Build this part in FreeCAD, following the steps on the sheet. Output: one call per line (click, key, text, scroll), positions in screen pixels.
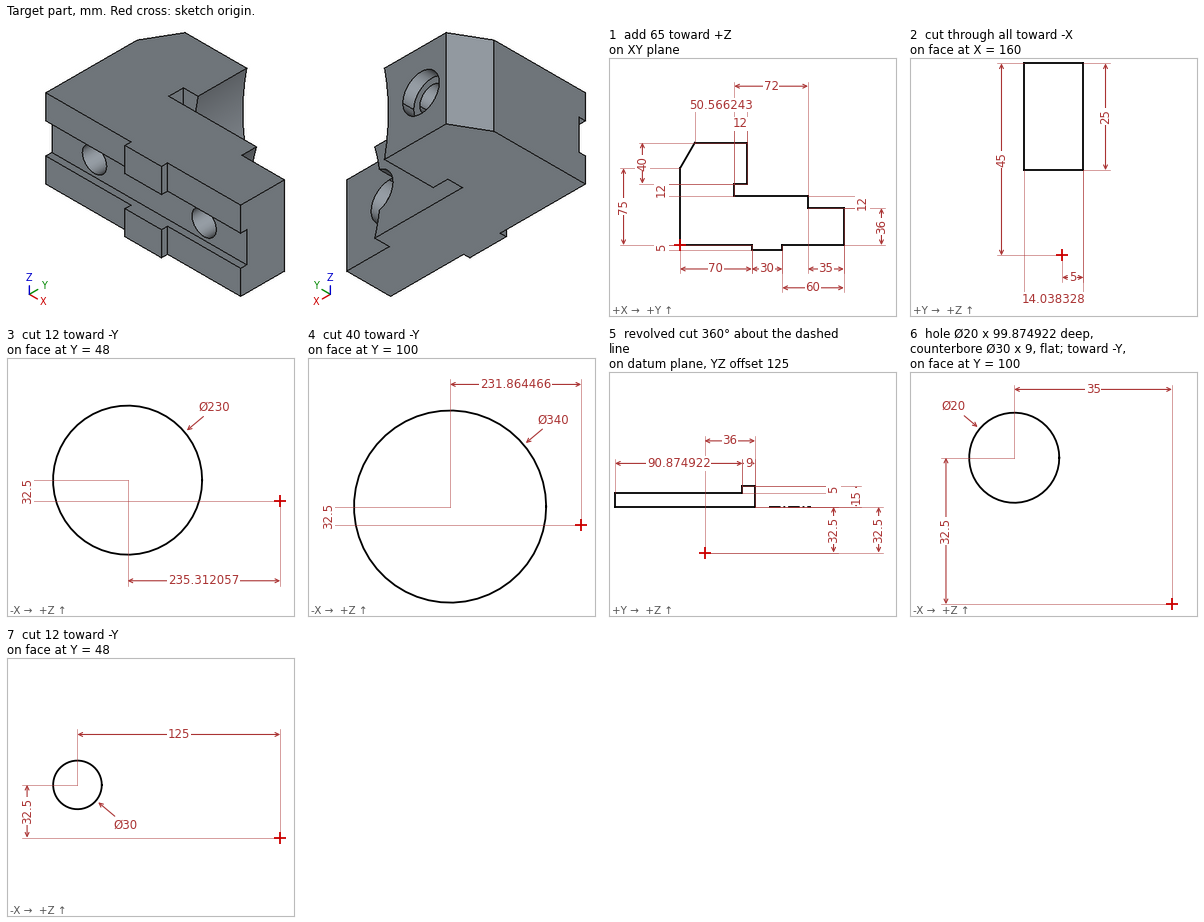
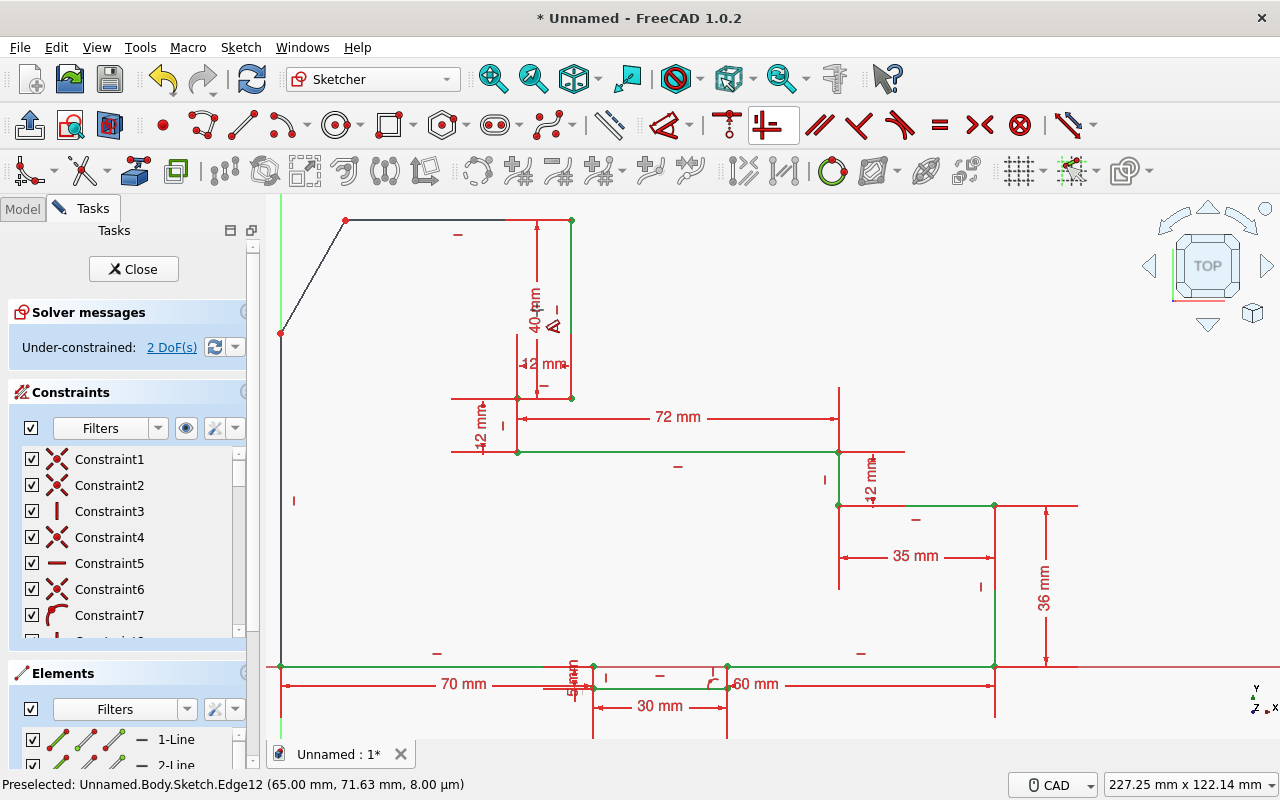
scroll(840, 491, down, 2)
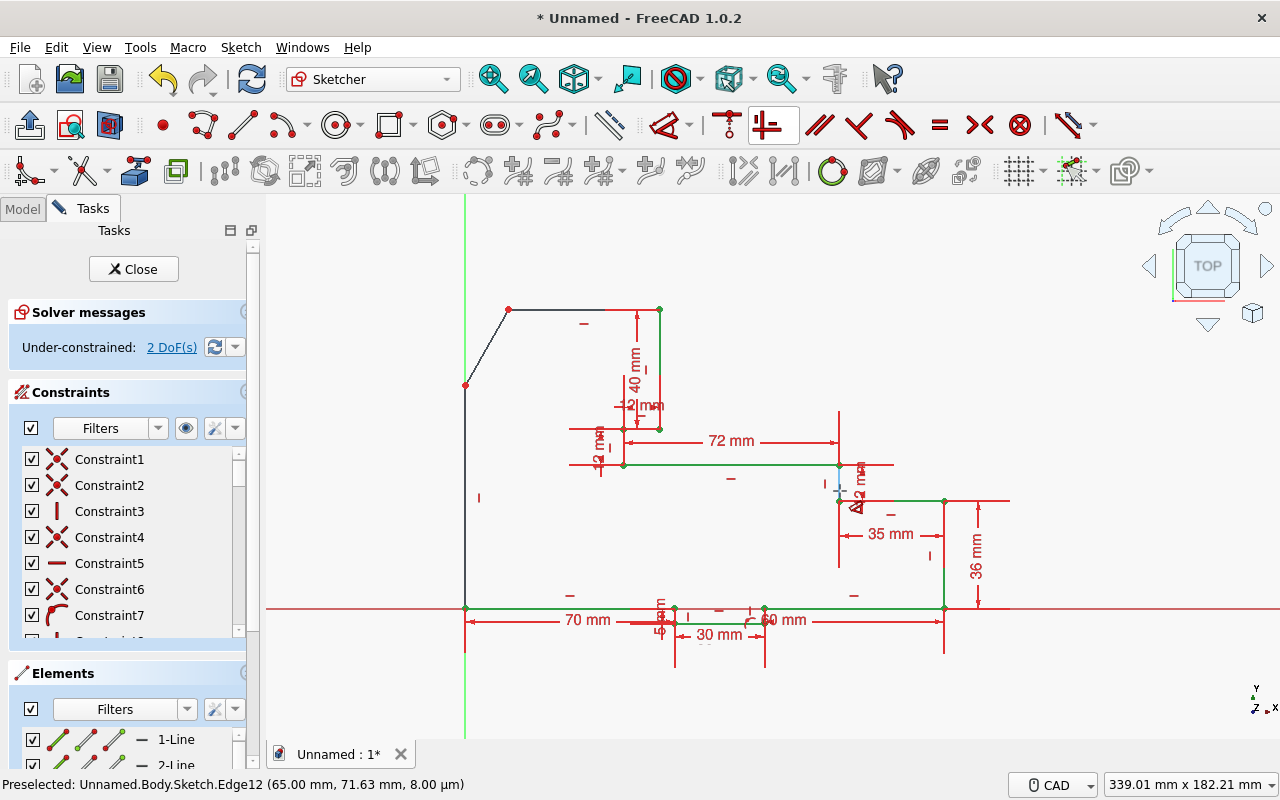
click(465, 453)
click(431, 497)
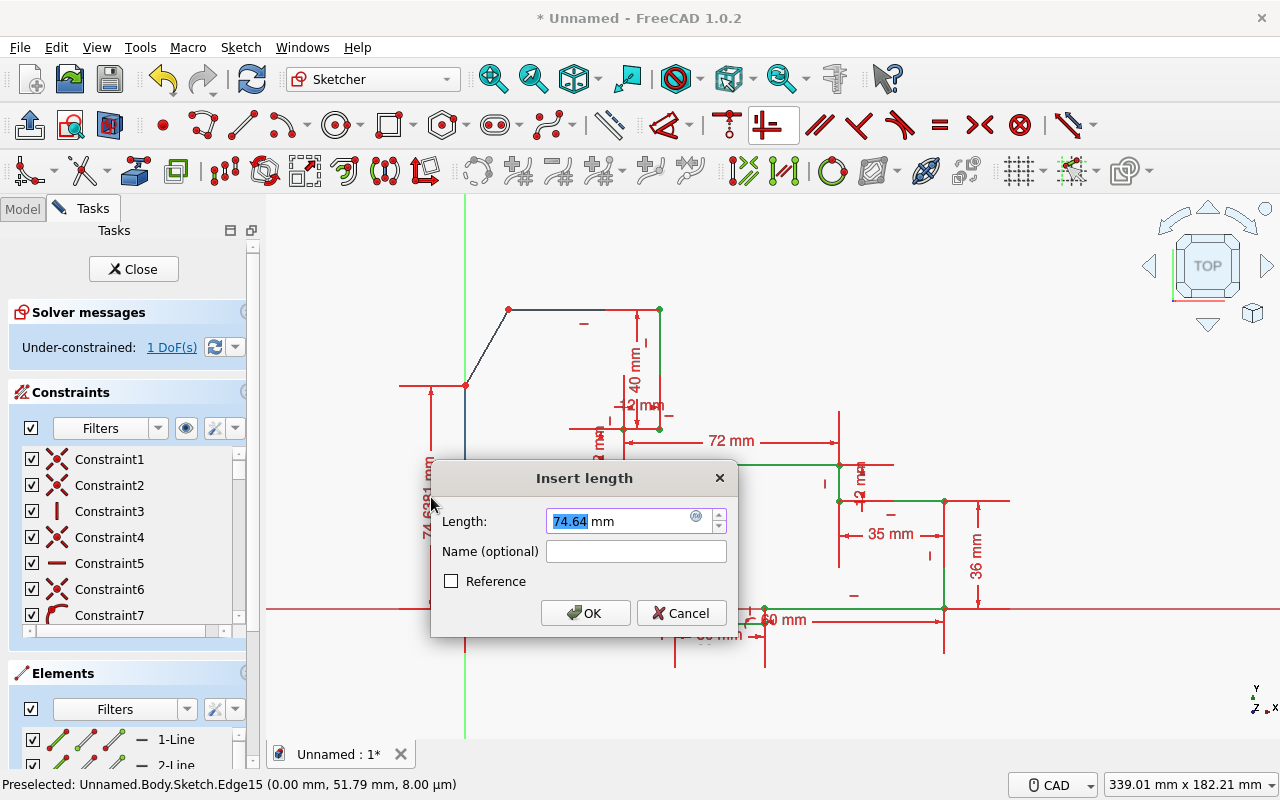
text(75)
key(Return)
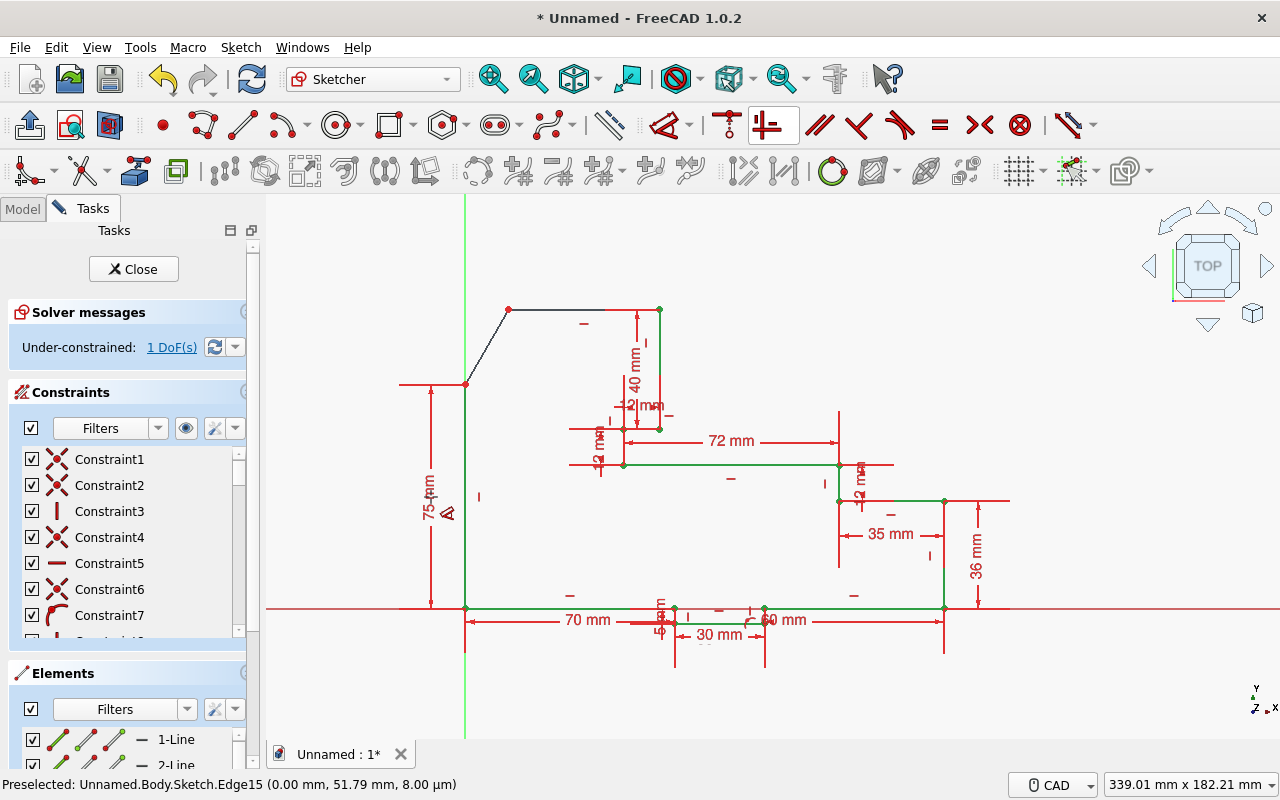
click(614, 310)
click(584, 276)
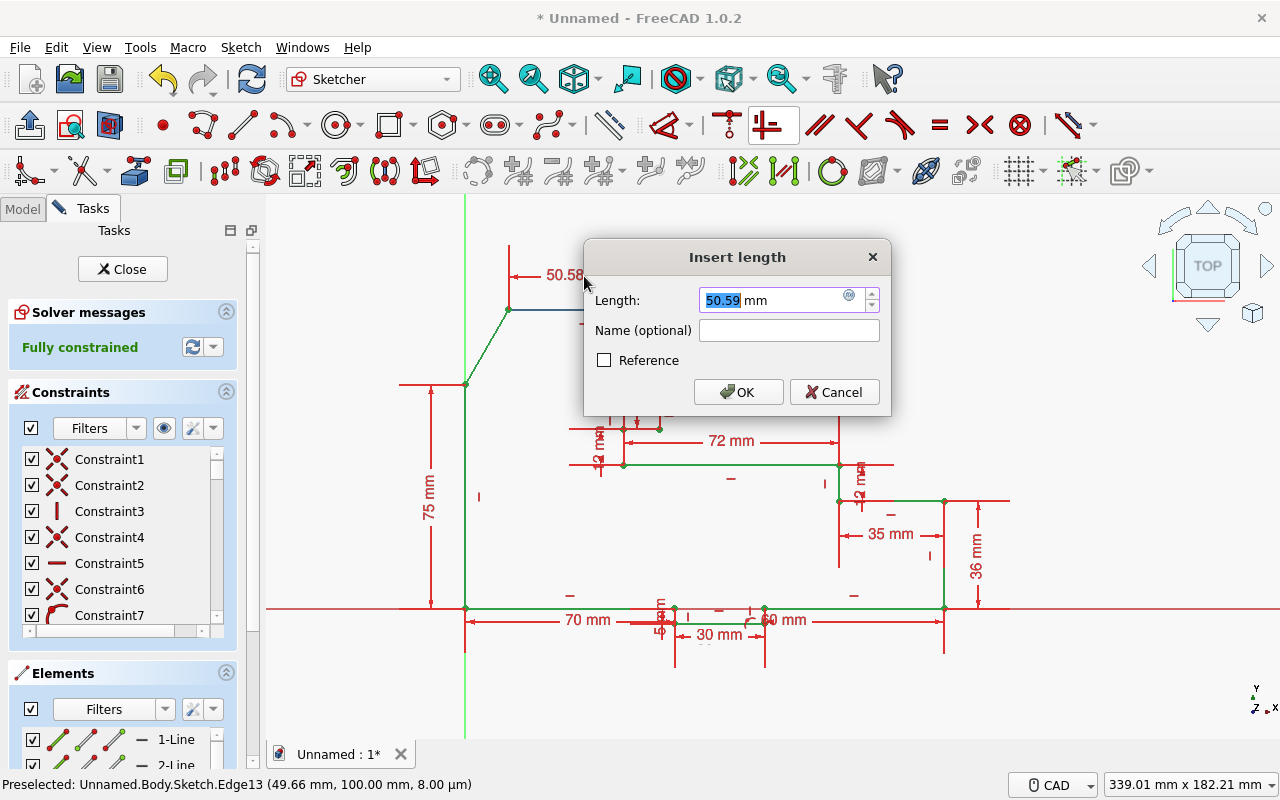
text(50.566243)
key(Return)
key(Escape)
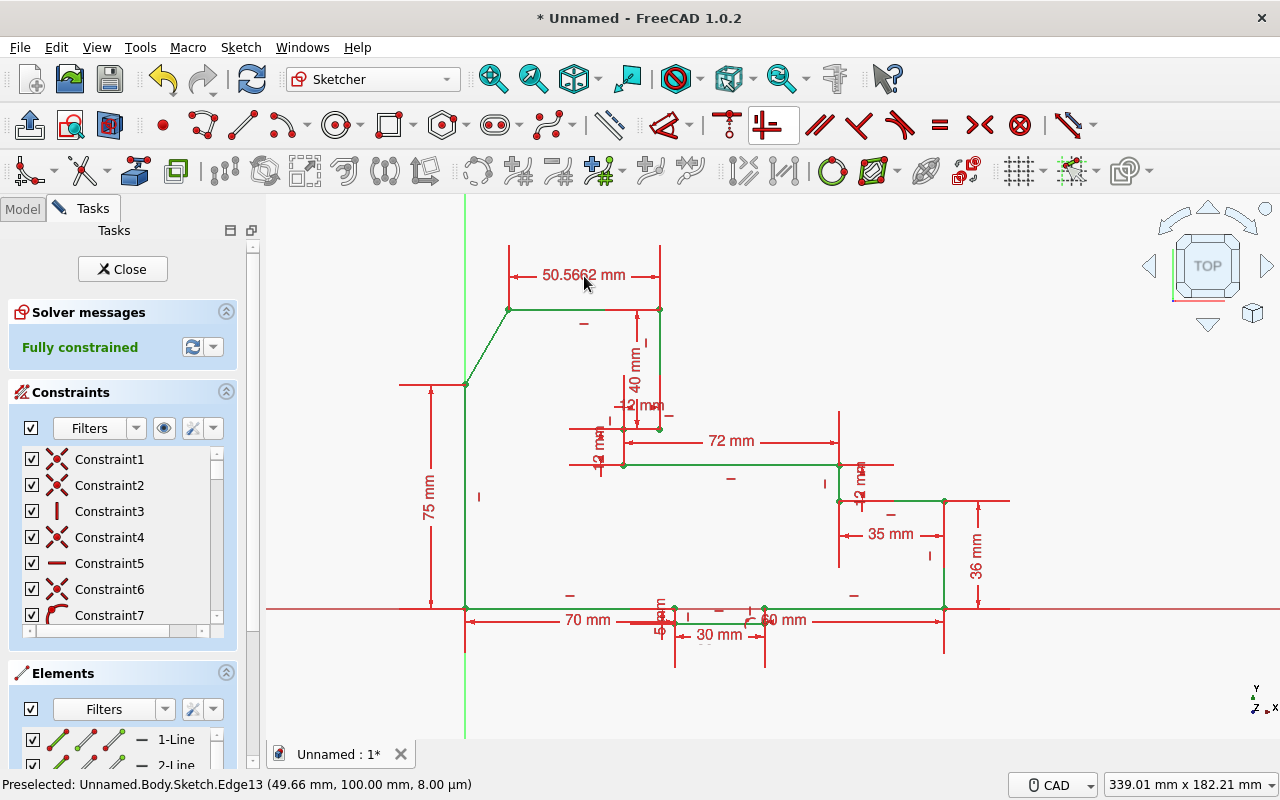
click(123, 269)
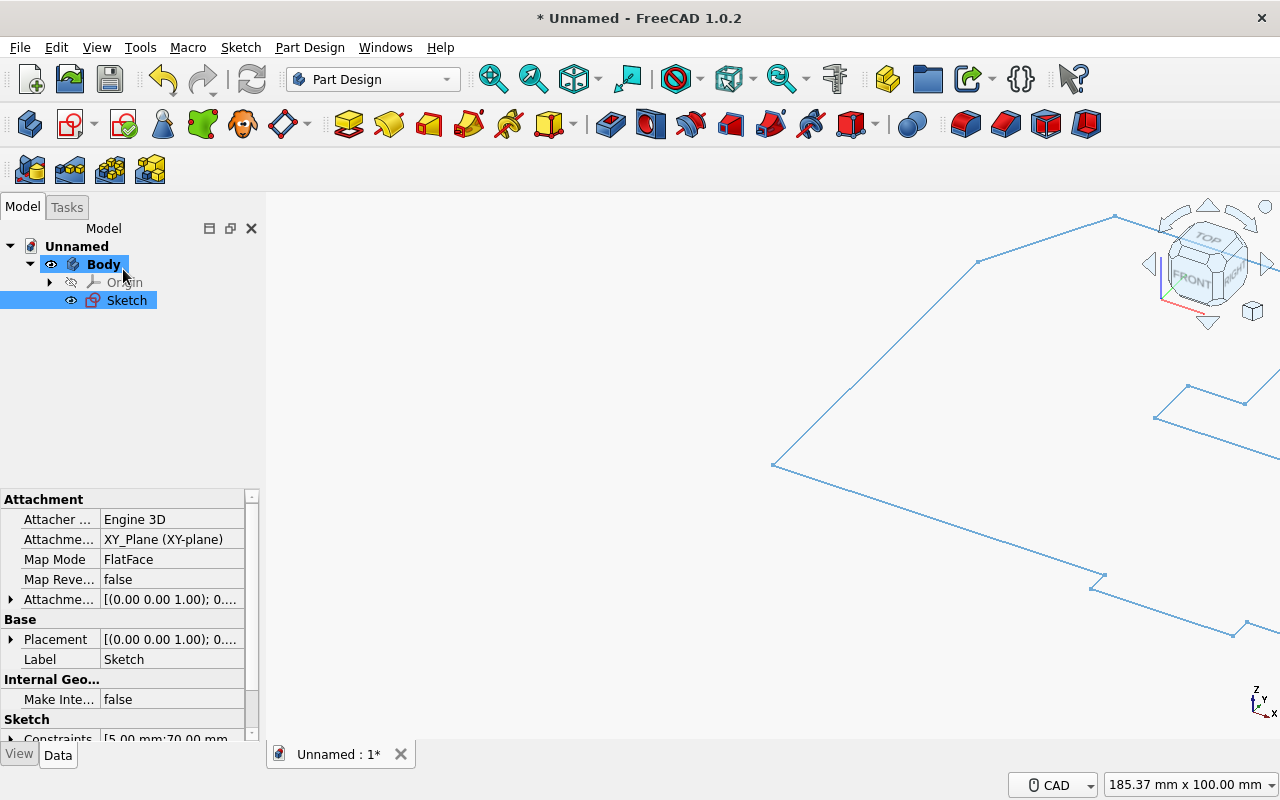
click(350, 124)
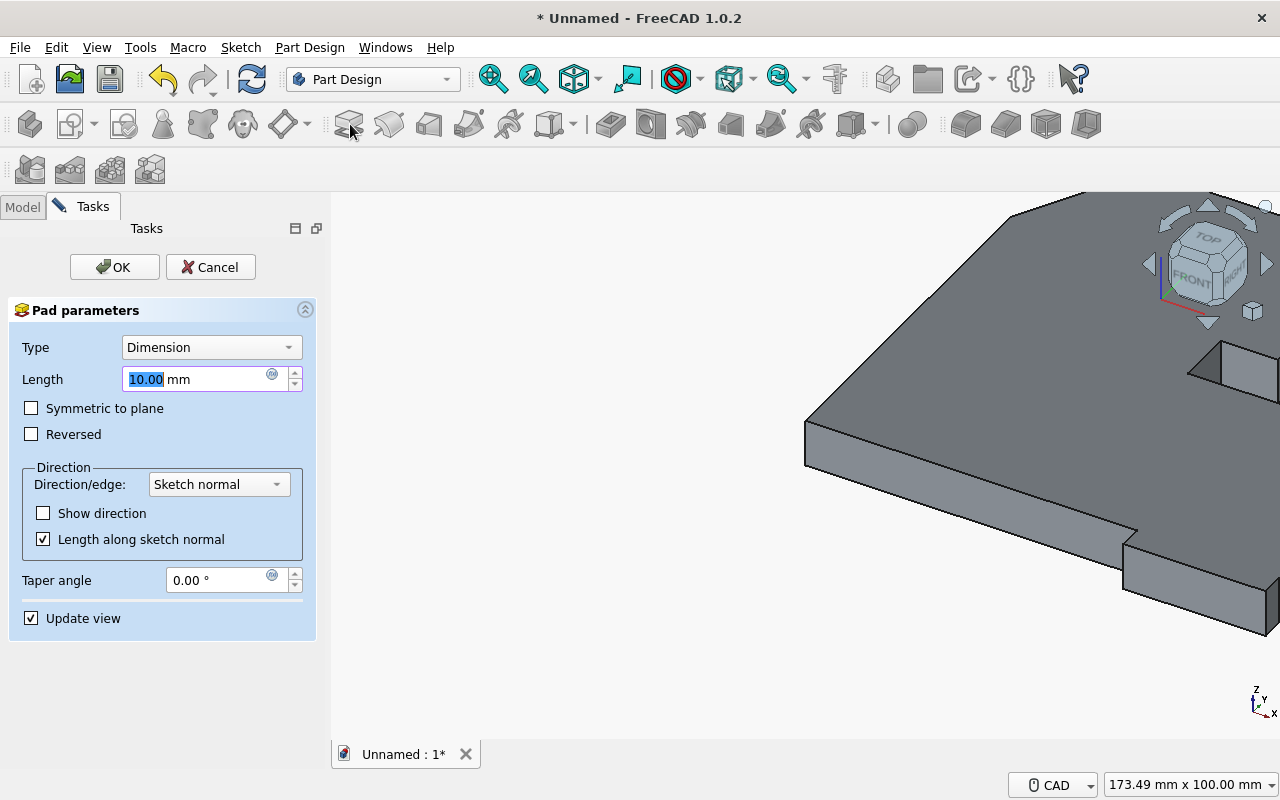
text(65)
key(Tab)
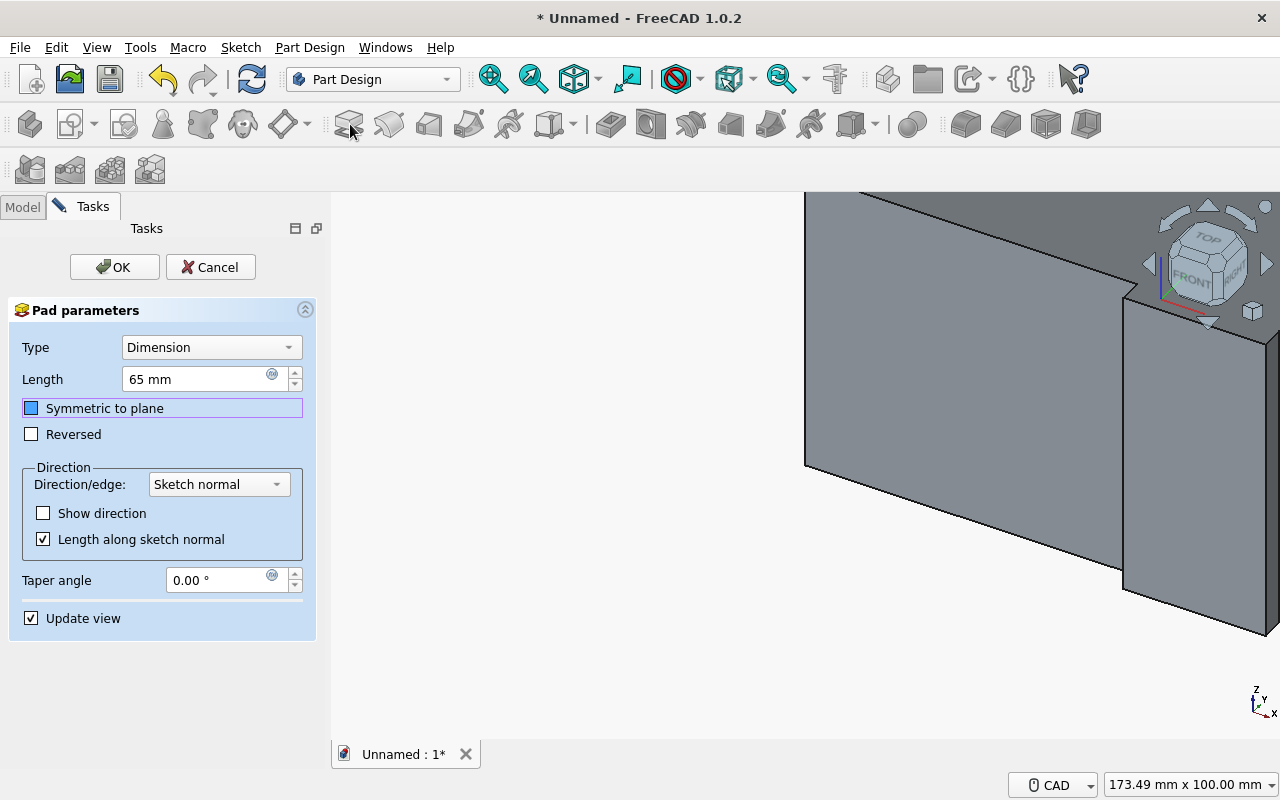
click(115, 267)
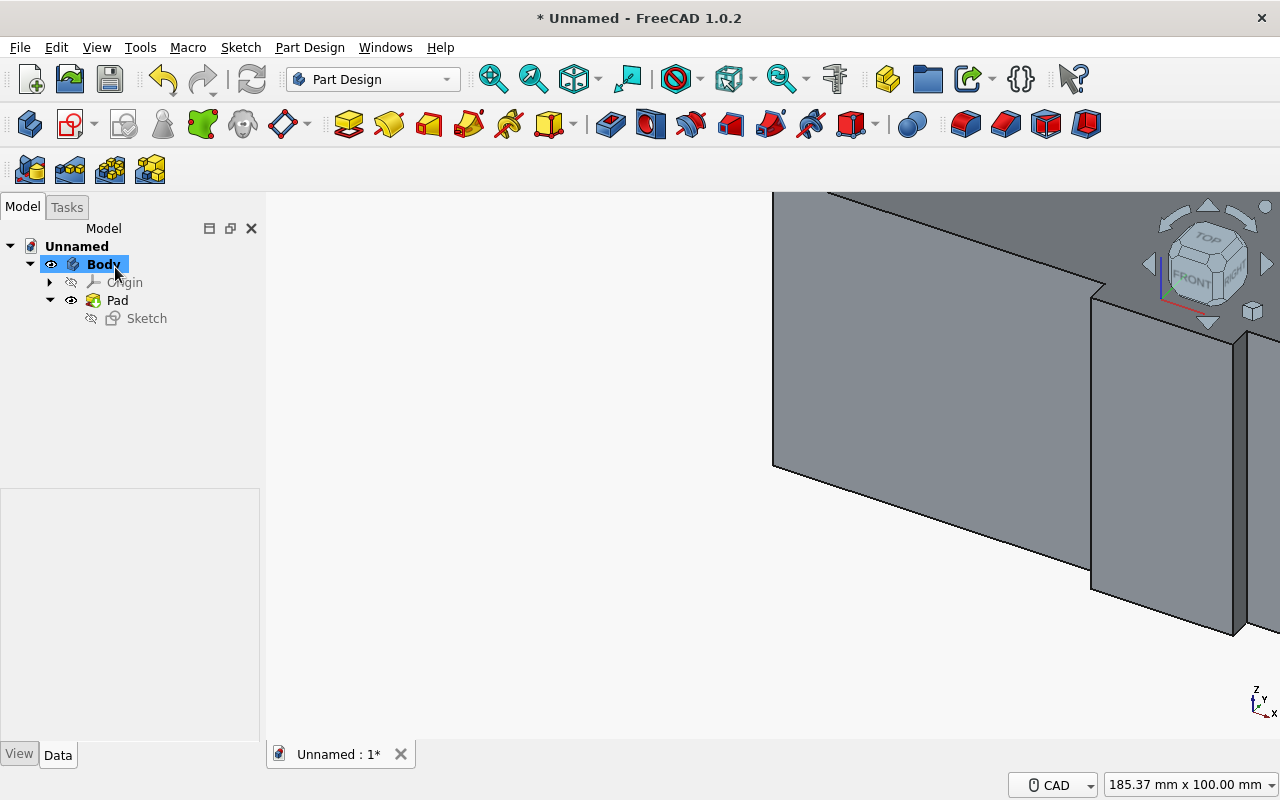
click(494, 80)